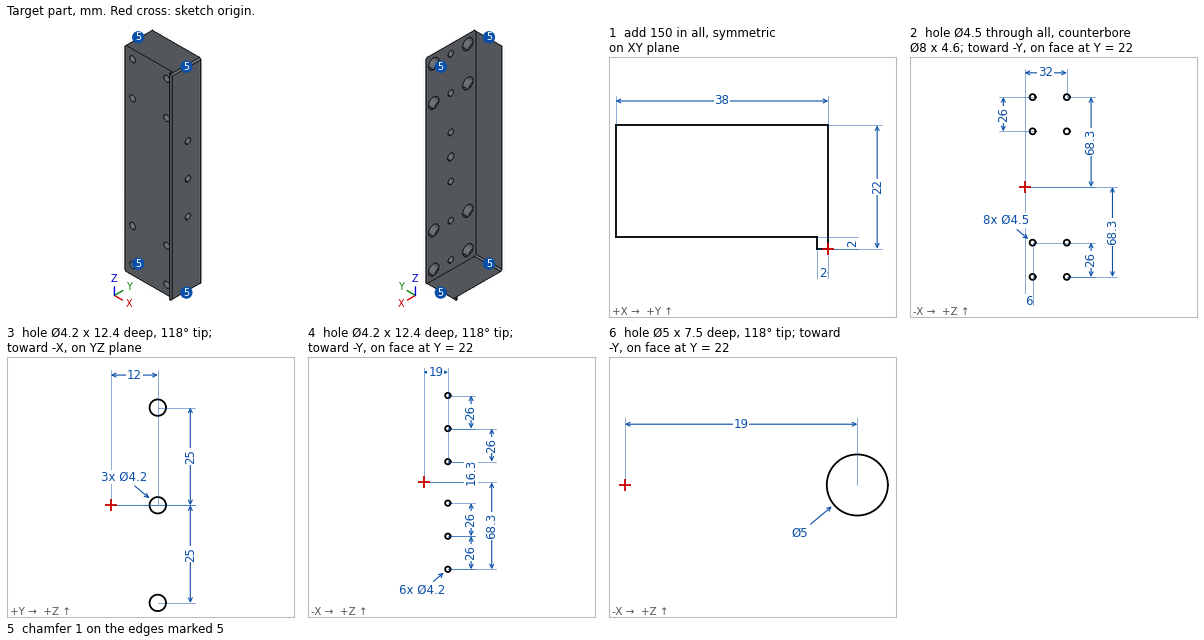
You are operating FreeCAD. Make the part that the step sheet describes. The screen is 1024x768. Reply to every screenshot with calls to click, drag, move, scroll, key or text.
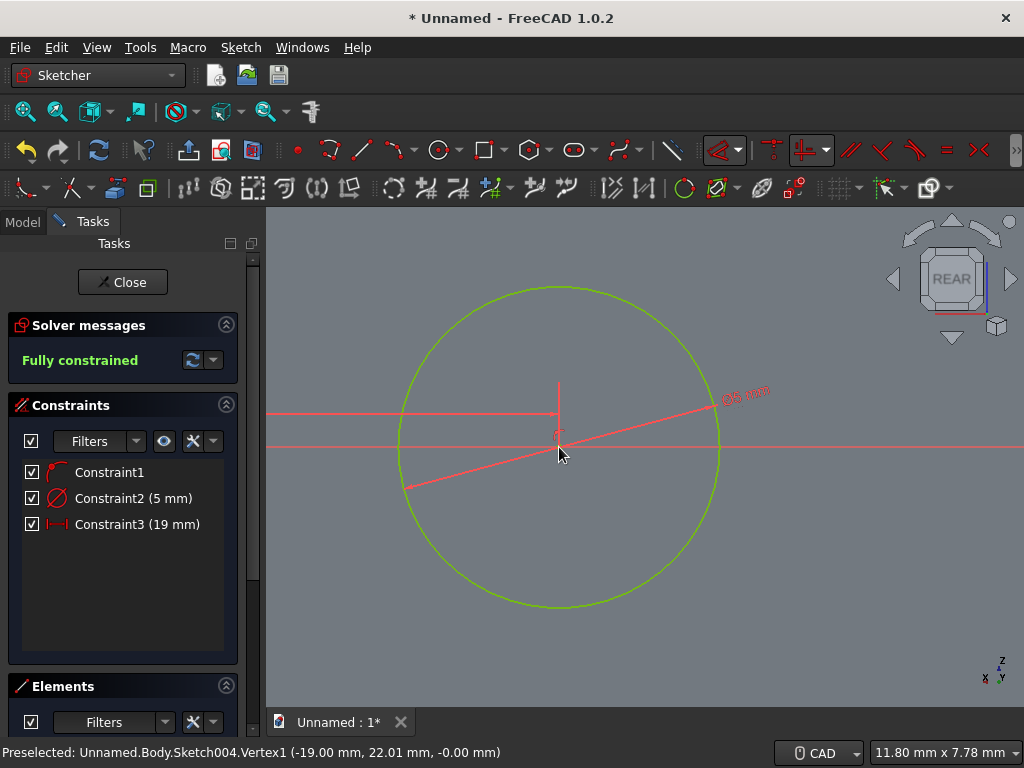
click(123, 282)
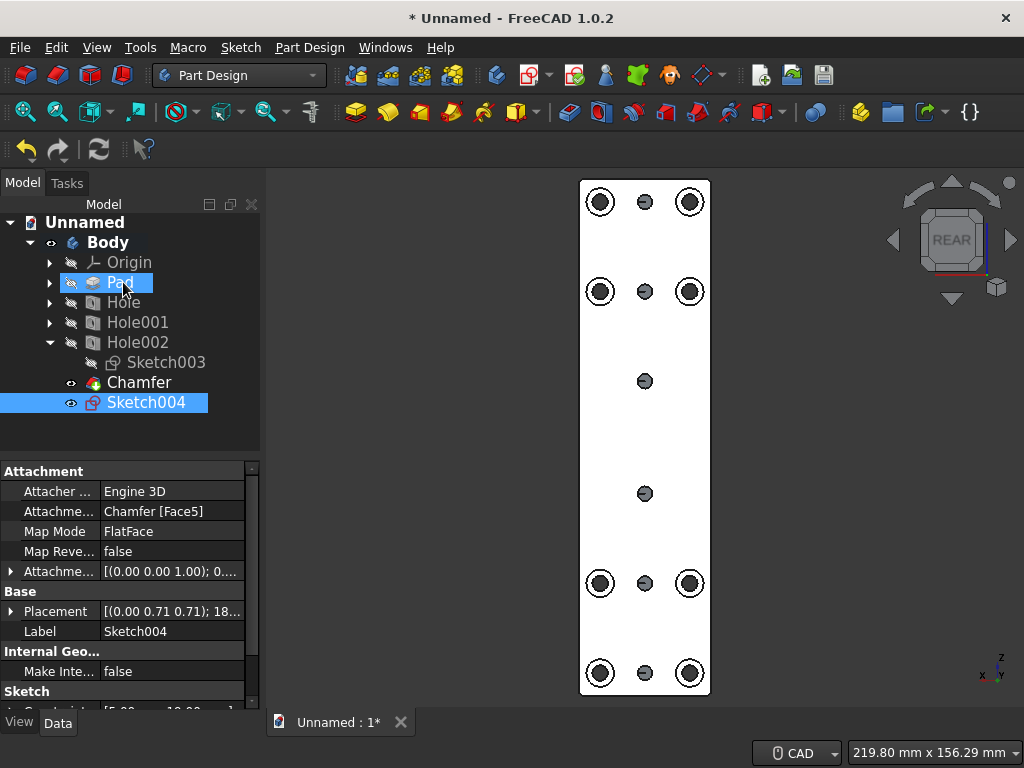
click(602, 112)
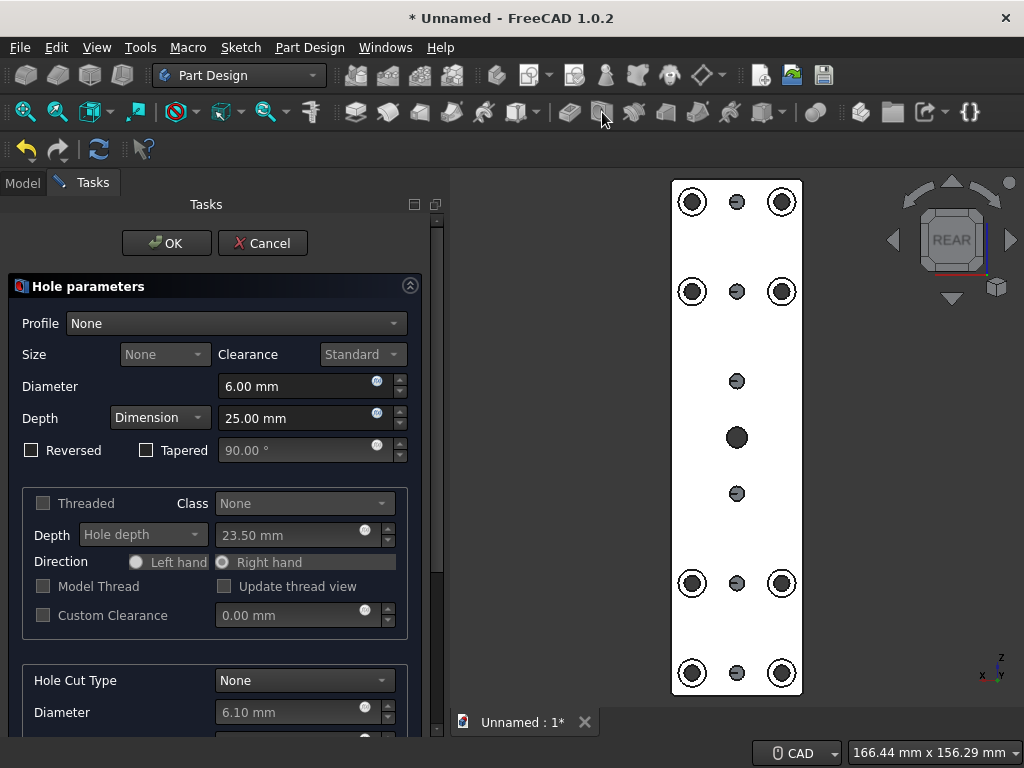
triple_click(305, 386)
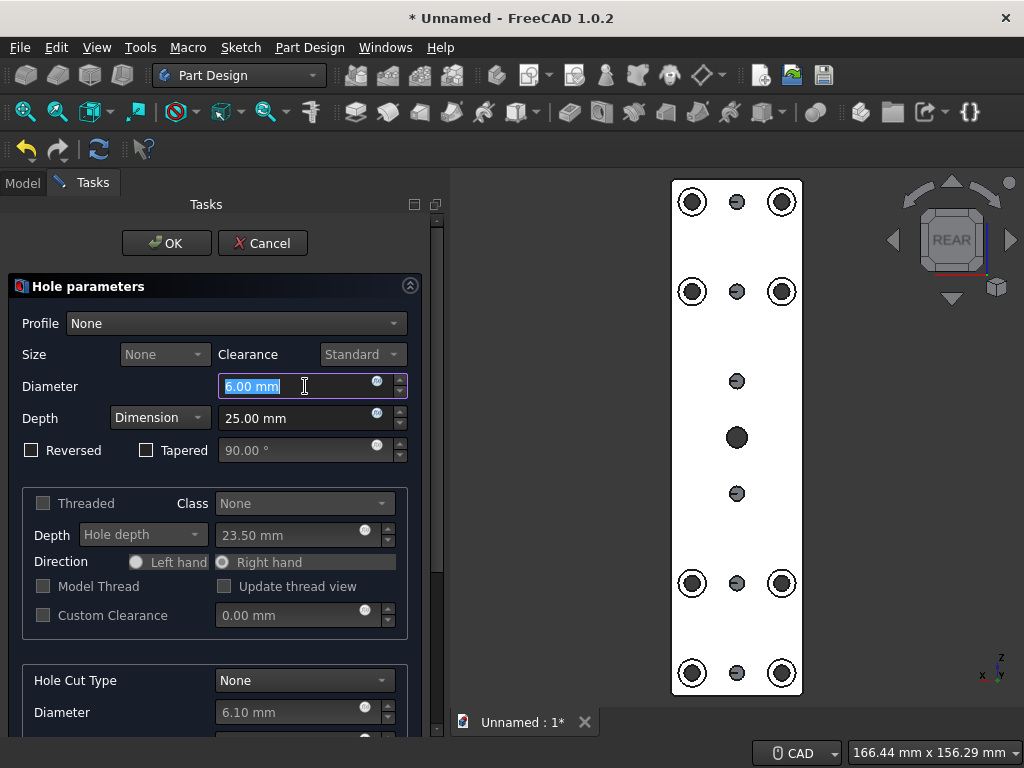
text(5)
key(Tab)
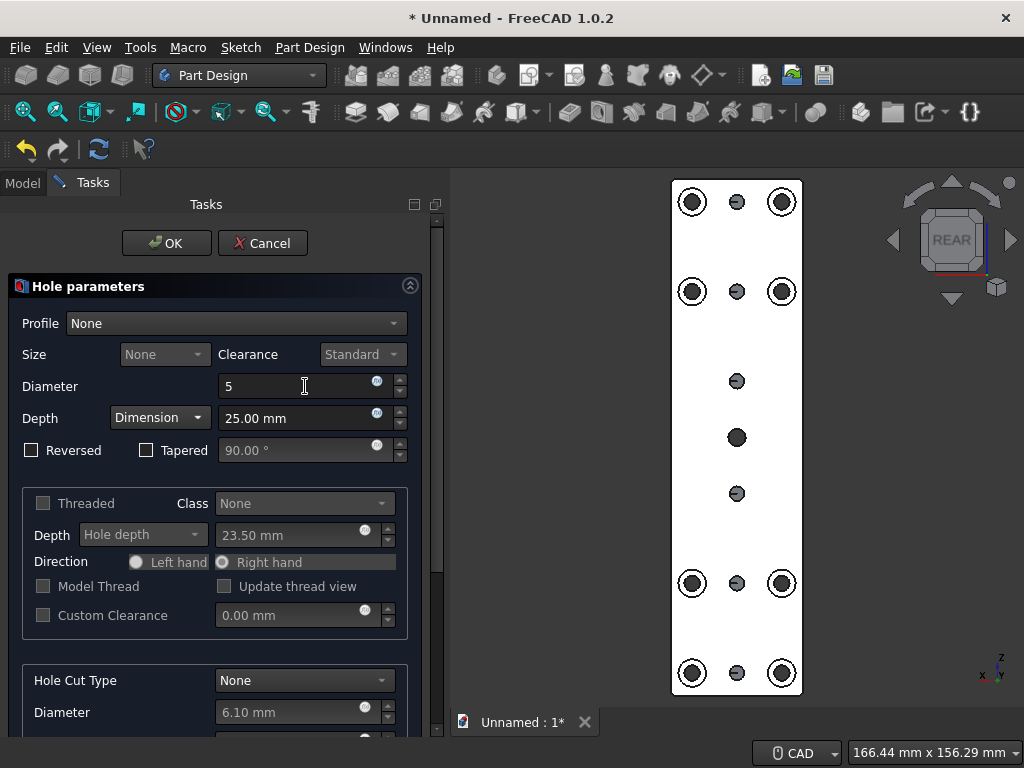
triple_click(305, 418)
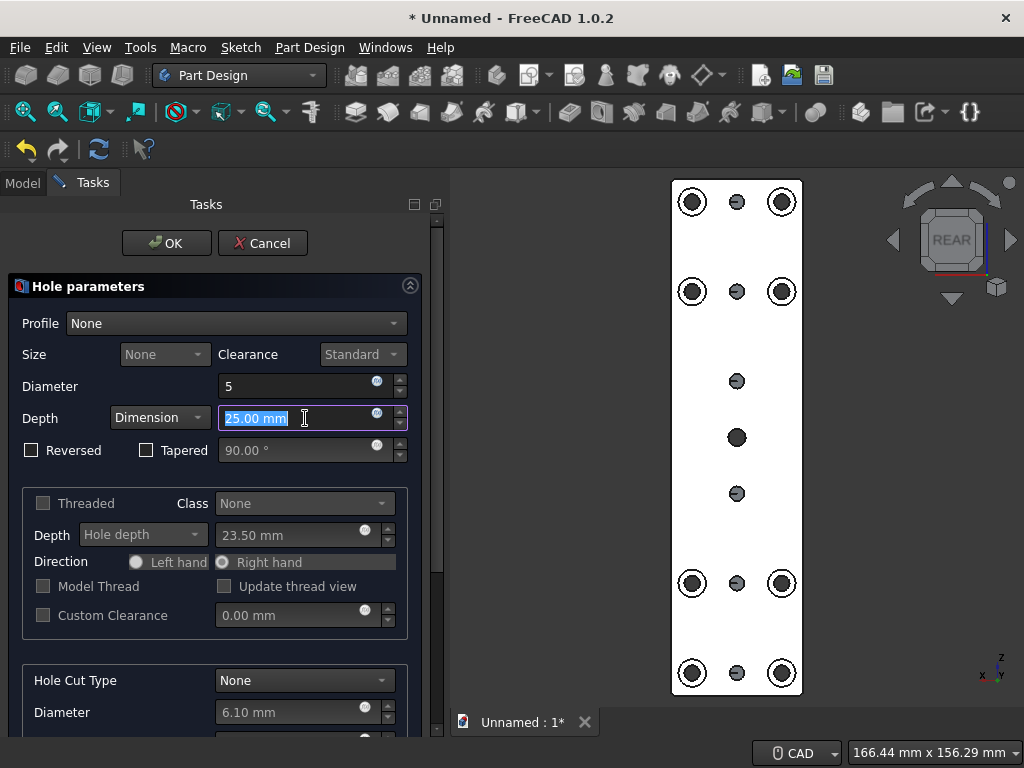
text(7.5)
key(Tab)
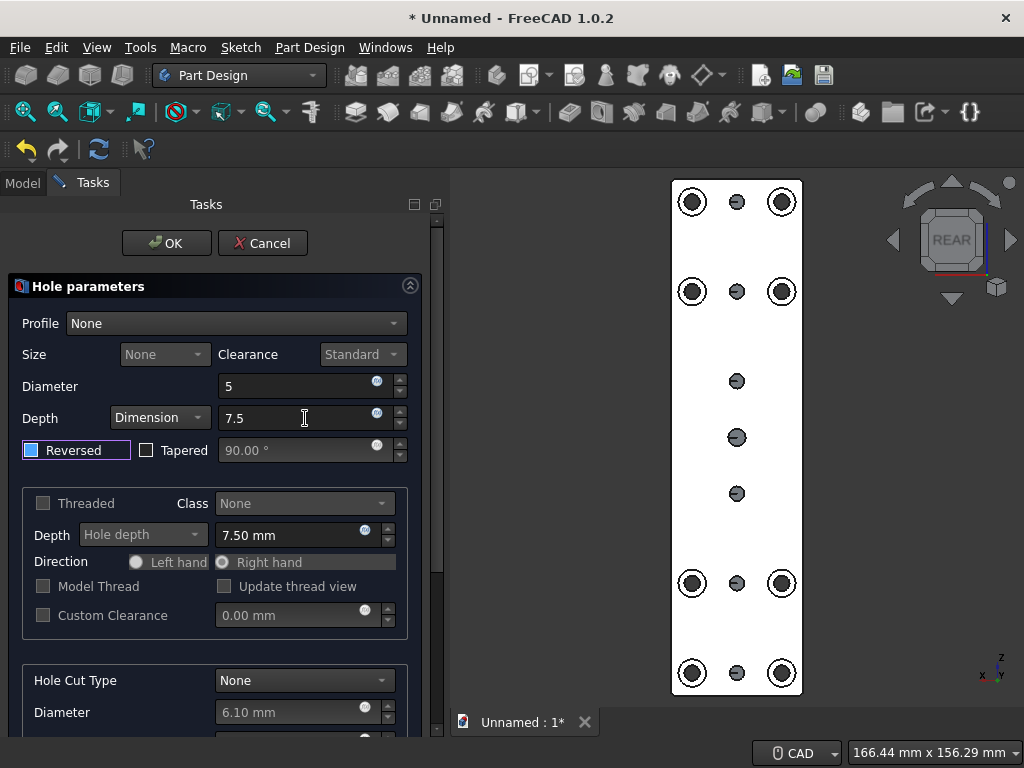
click(167, 243)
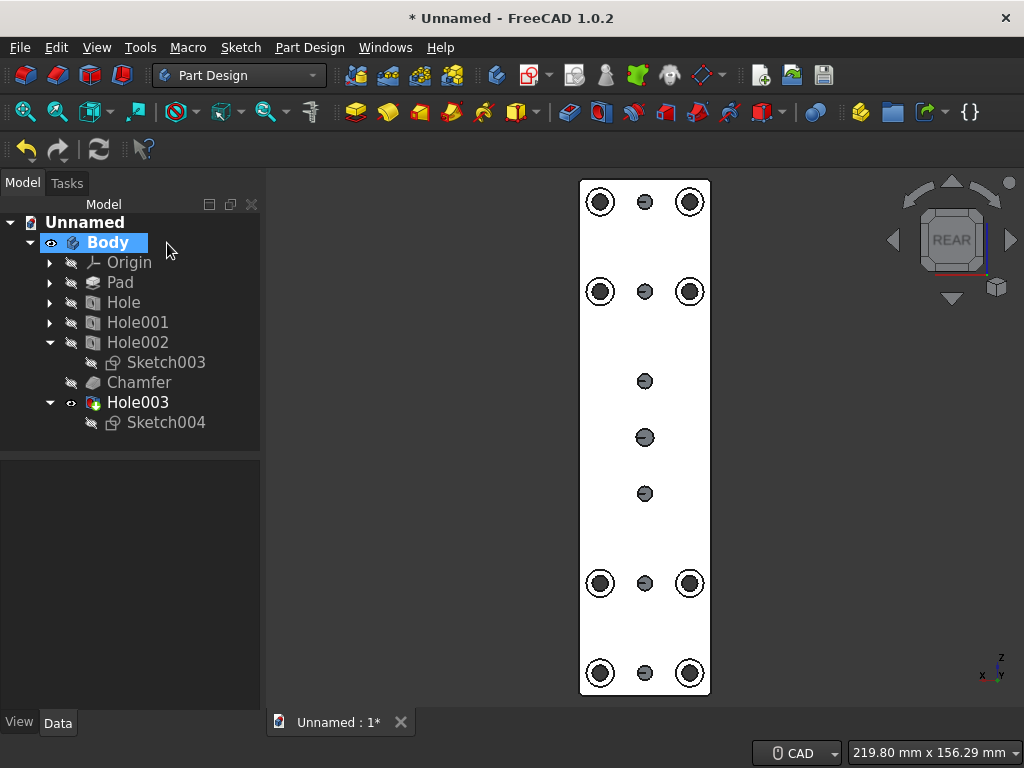
key(0)